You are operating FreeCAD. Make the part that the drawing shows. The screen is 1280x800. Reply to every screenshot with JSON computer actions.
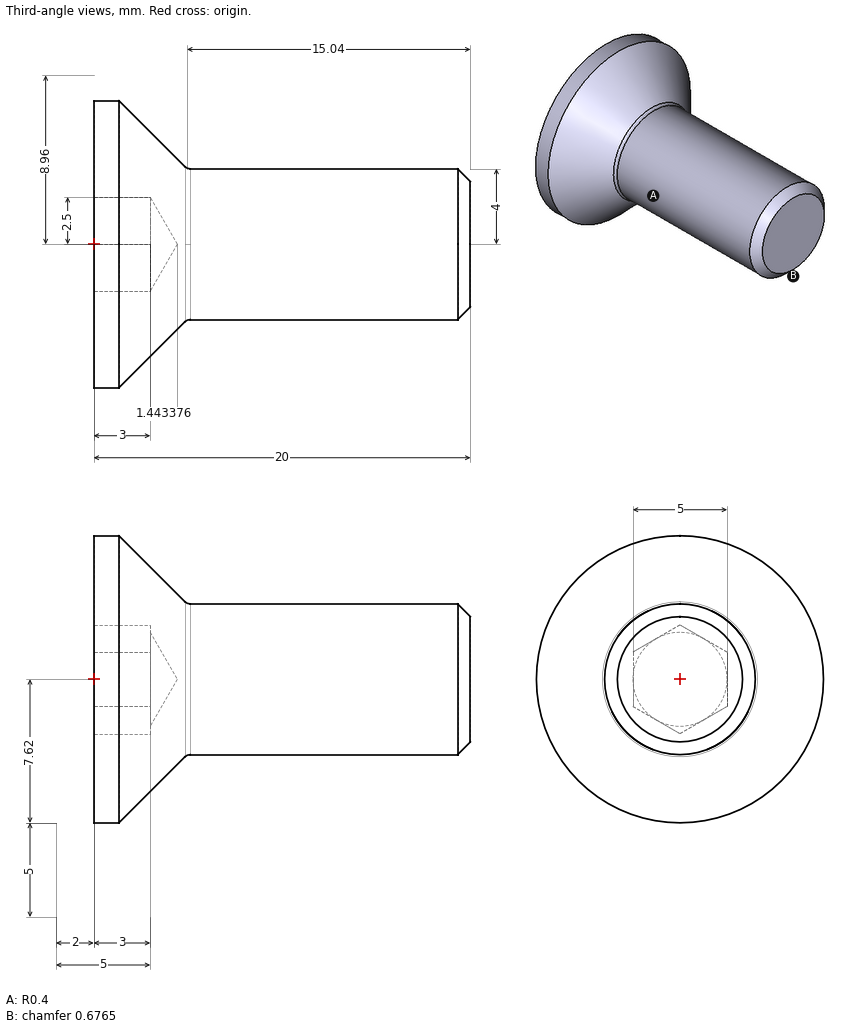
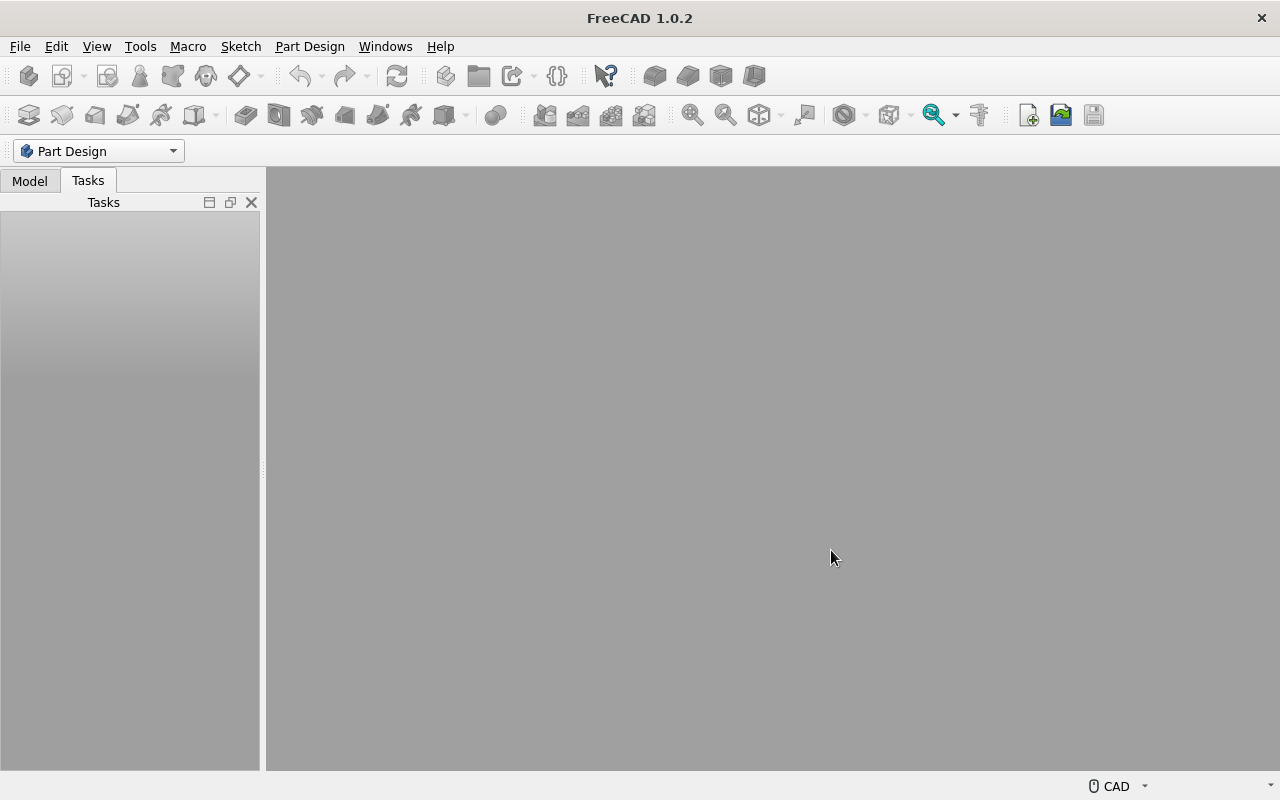
{"action": "left_click", "coordinate": [1028, 116]}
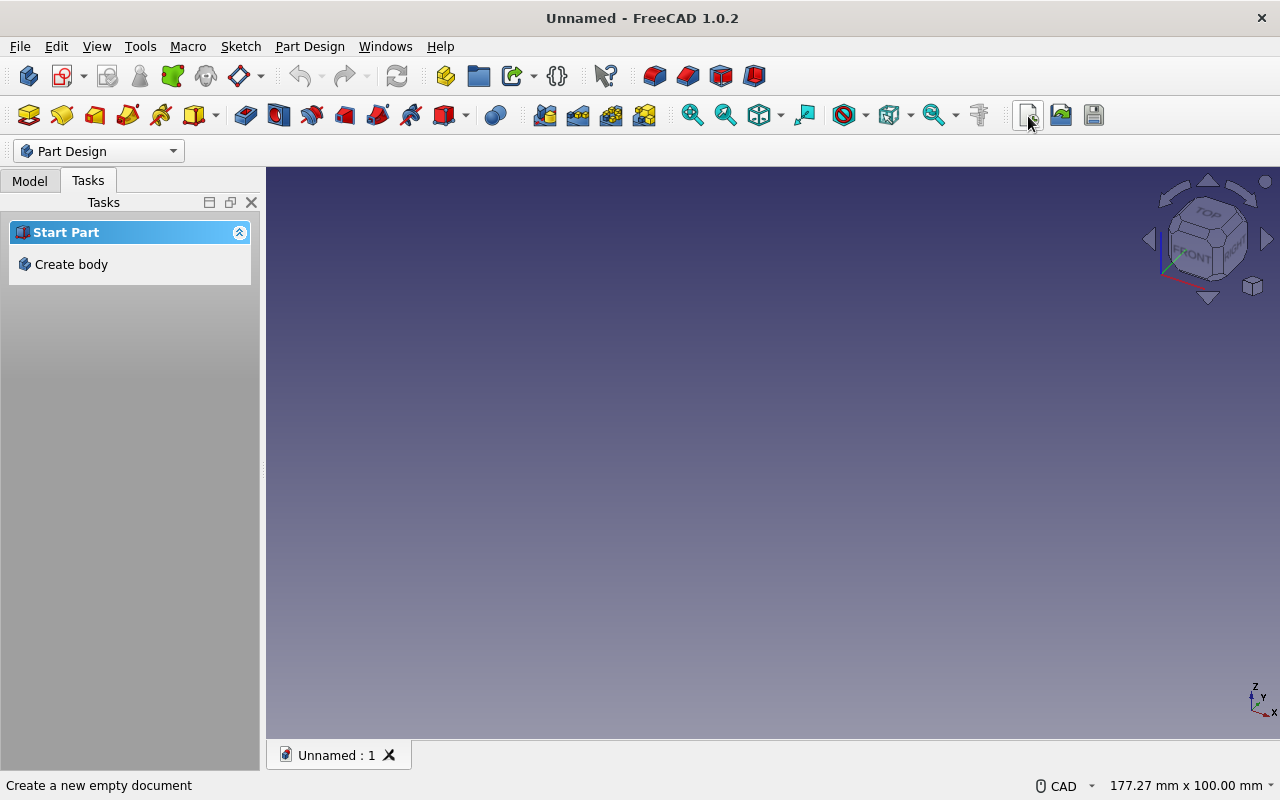
{"action": "left_click", "coordinate": [62, 76]}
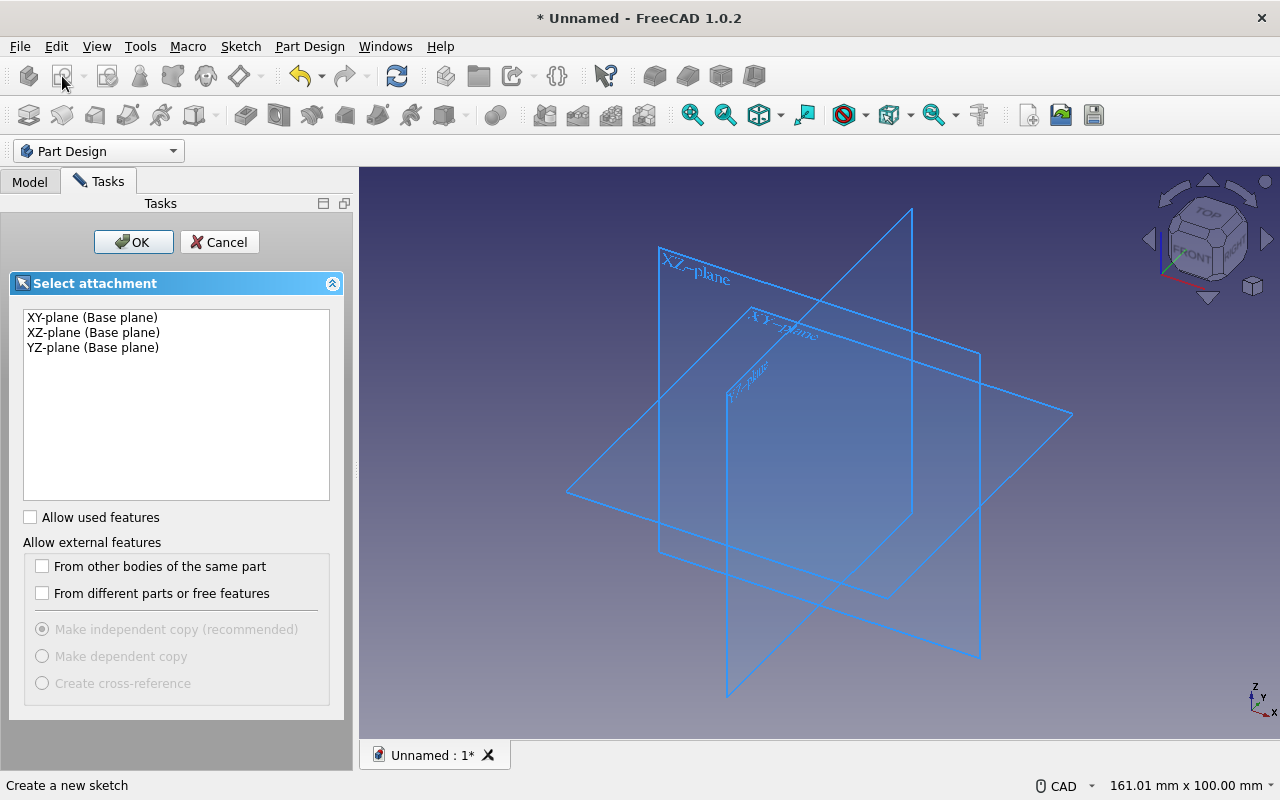
{"action": "left_click", "coordinate": [84, 318]}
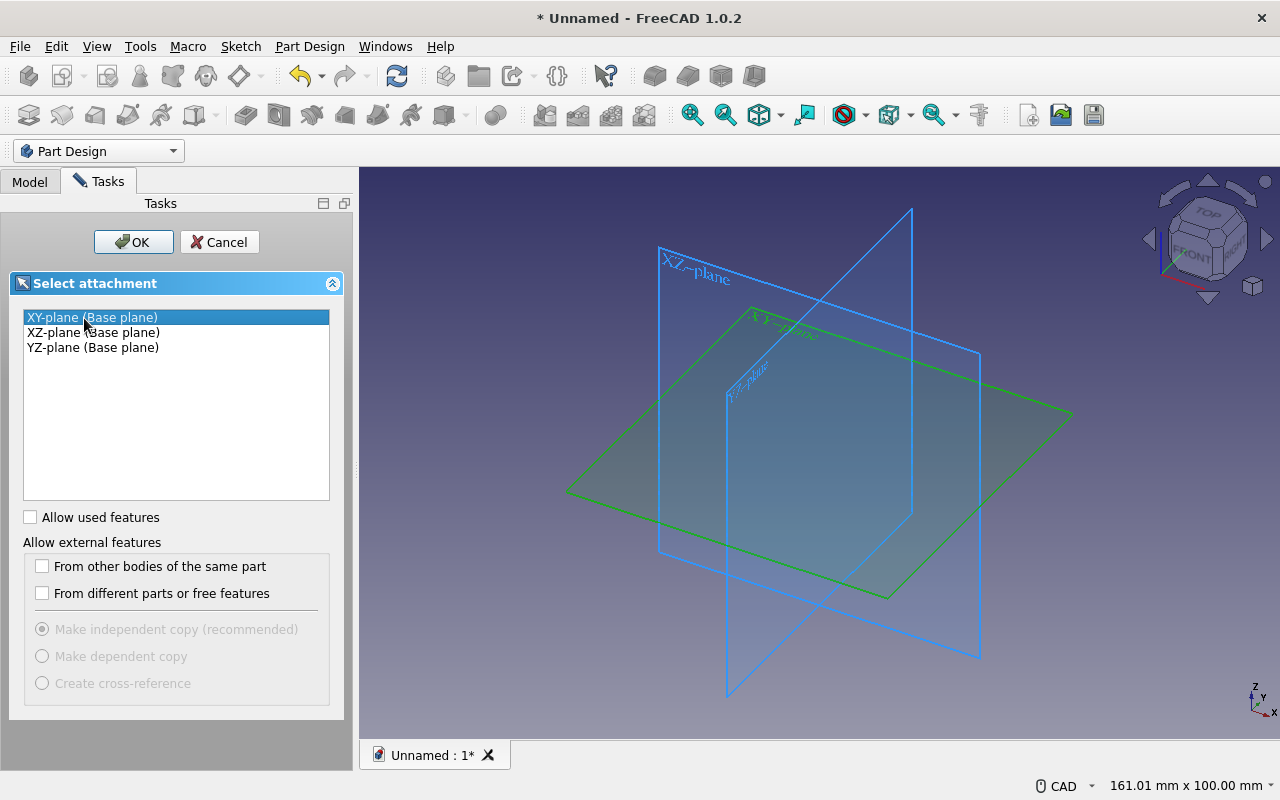
{"action": "left_click", "coordinate": [134, 242]}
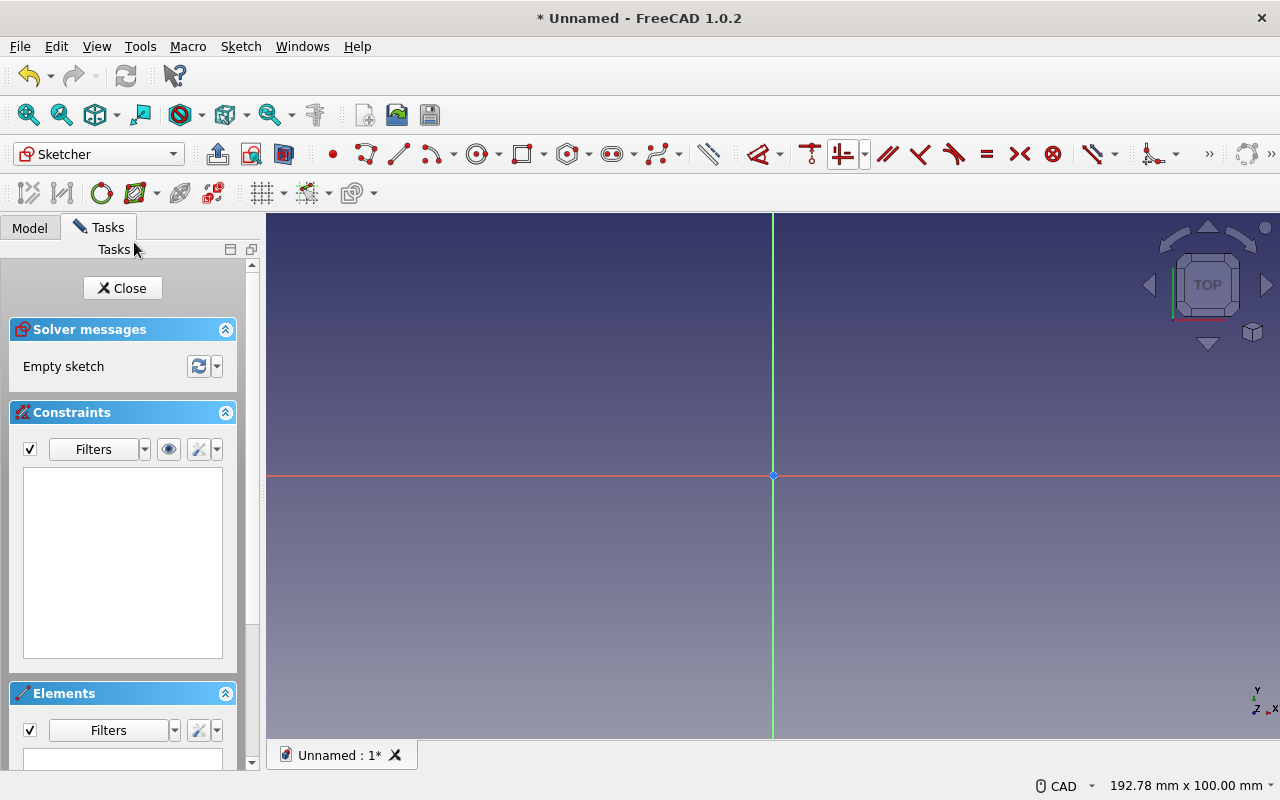
{"action": "scroll", "coordinate": [850, 448], "scroll_direction": "up", "scroll_amount": 9}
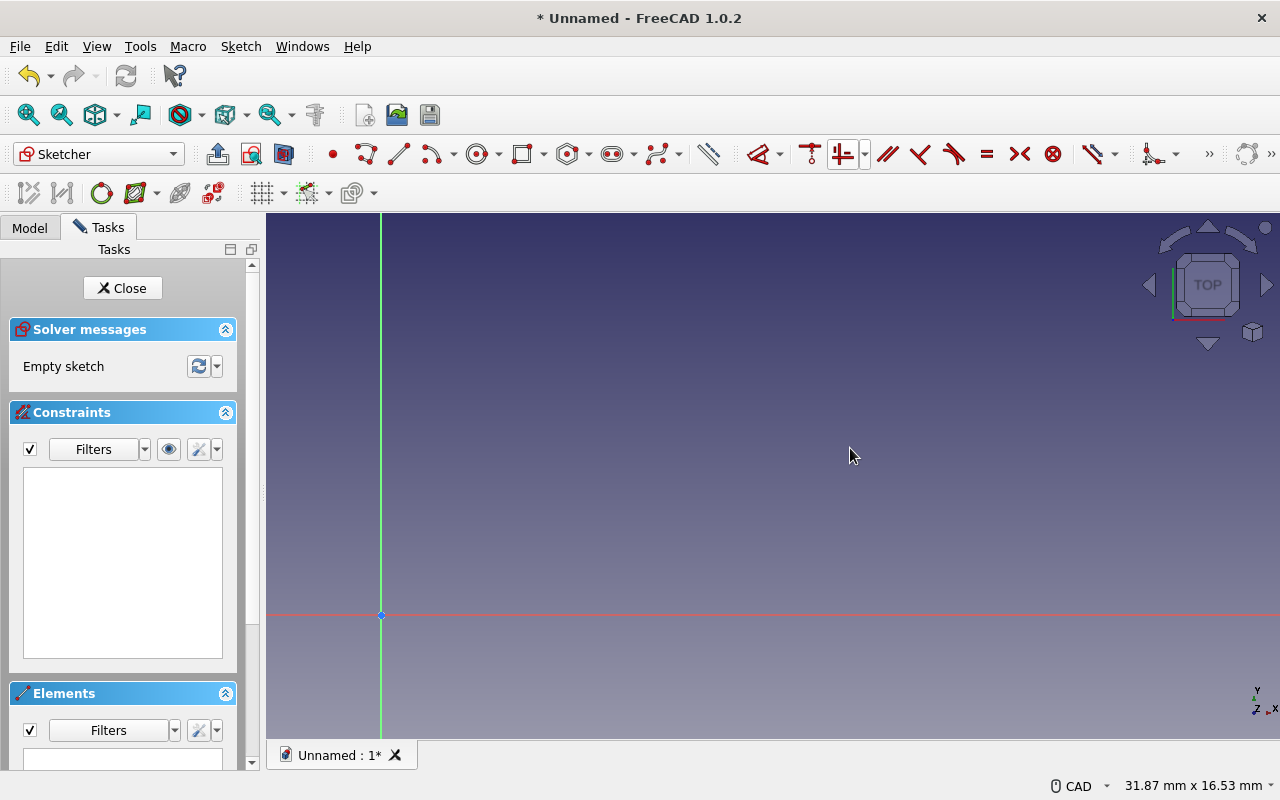
{"action": "left_click", "coordinate": [366, 154]}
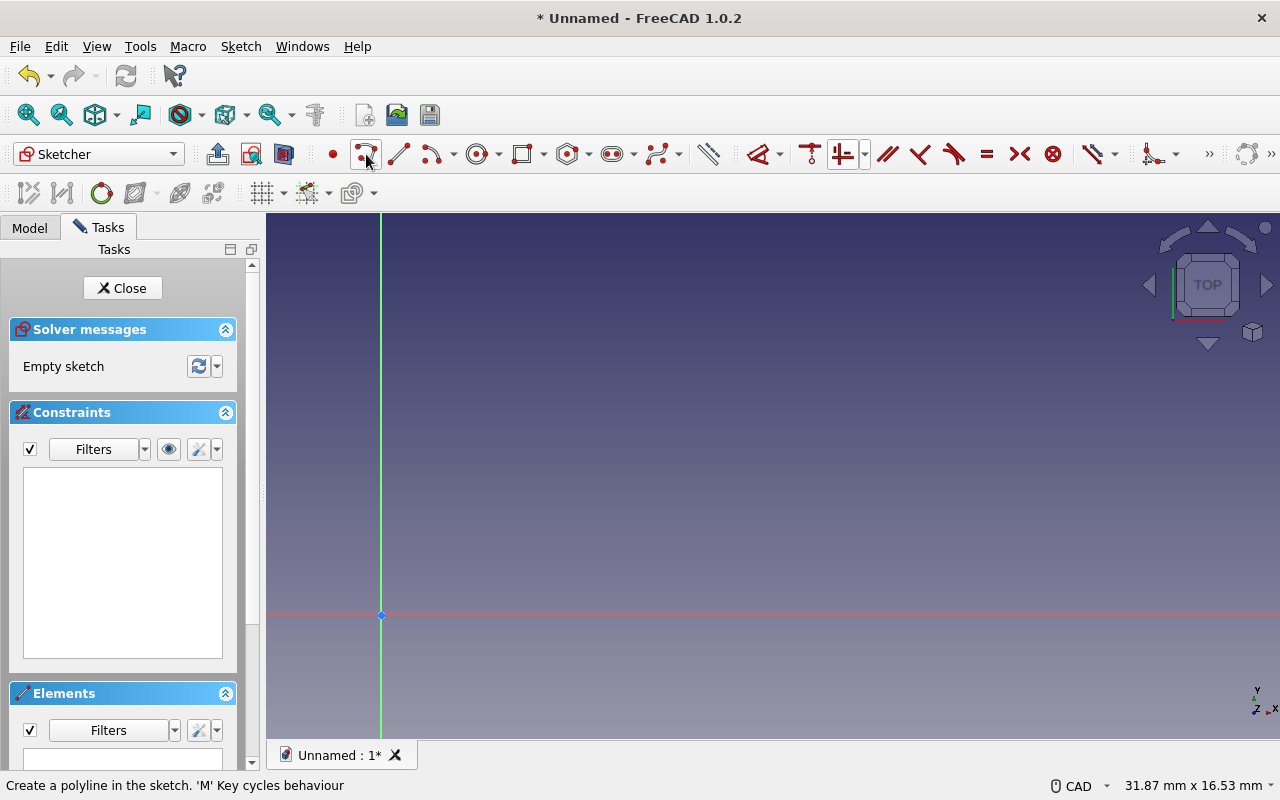
{"action": "left_click", "coordinate": [381, 615]}
{"action": "left_click", "coordinate": [1018, 606]}
{"action": "left_click", "coordinate": [1018, 488]}
{"action": "left_click", "coordinate": [539, 488]}
{"action": "left_click", "coordinate": [390, 330]}
{"action": "left_click", "coordinate": [381, 615]}
{"action": "key", "text": "Escape"}
{"action": "key", "text": "Escape"}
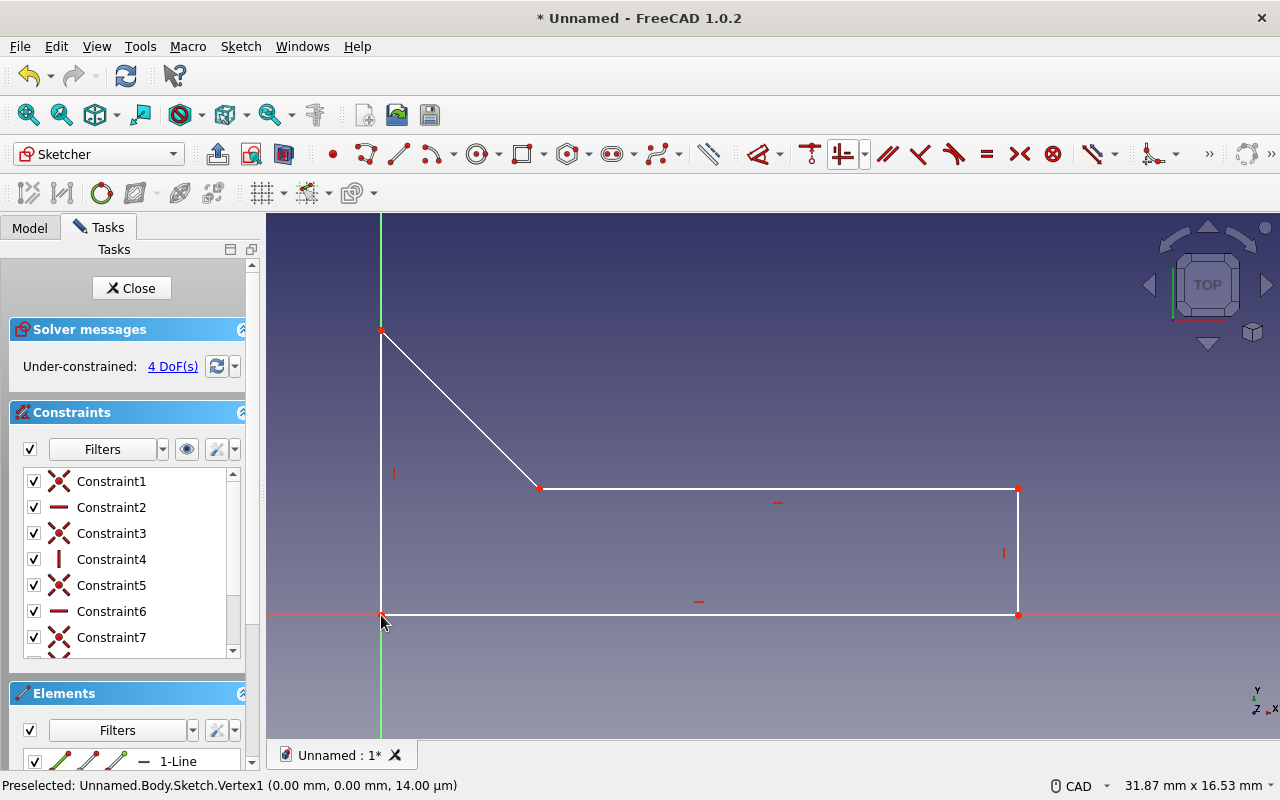
{"action": "left_click", "coordinate": [758, 154]}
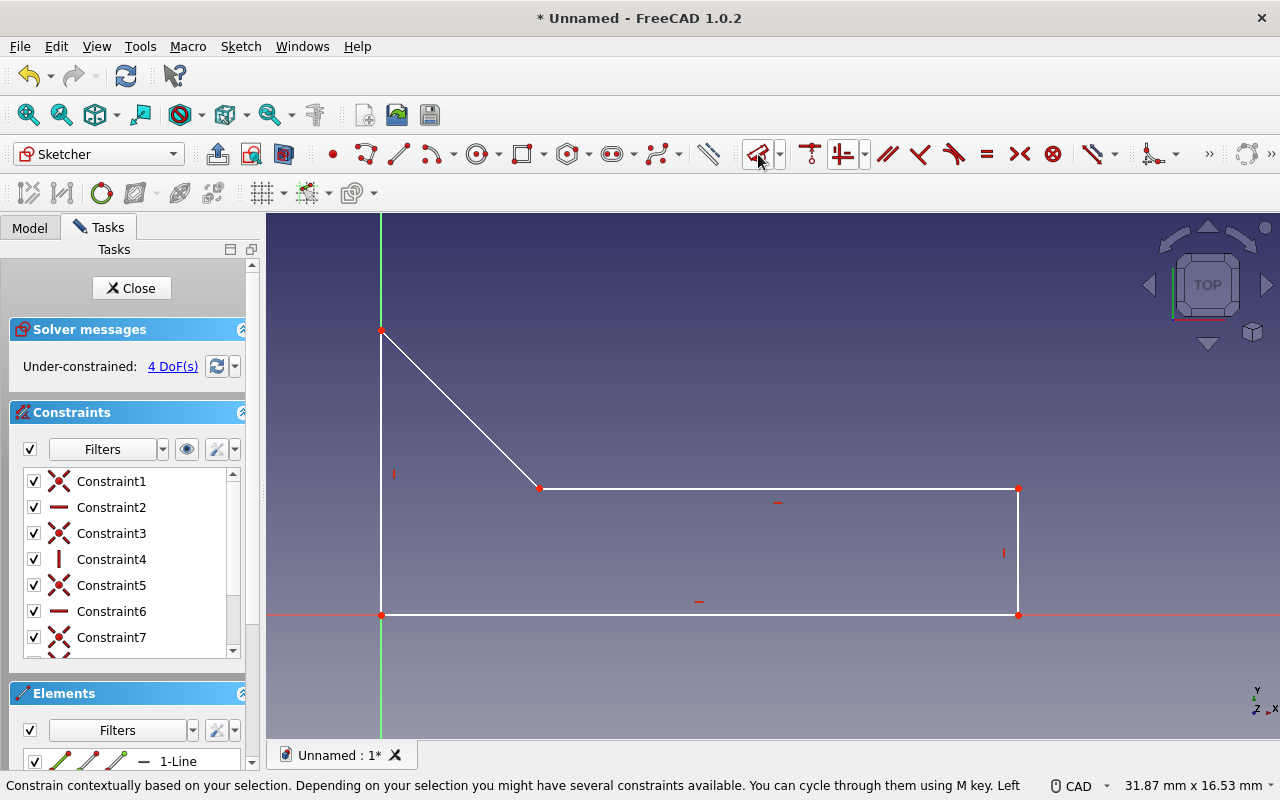
{"action": "left_click", "coordinate": [1018, 577]}
{"action": "left_click", "coordinate": [1052, 552]}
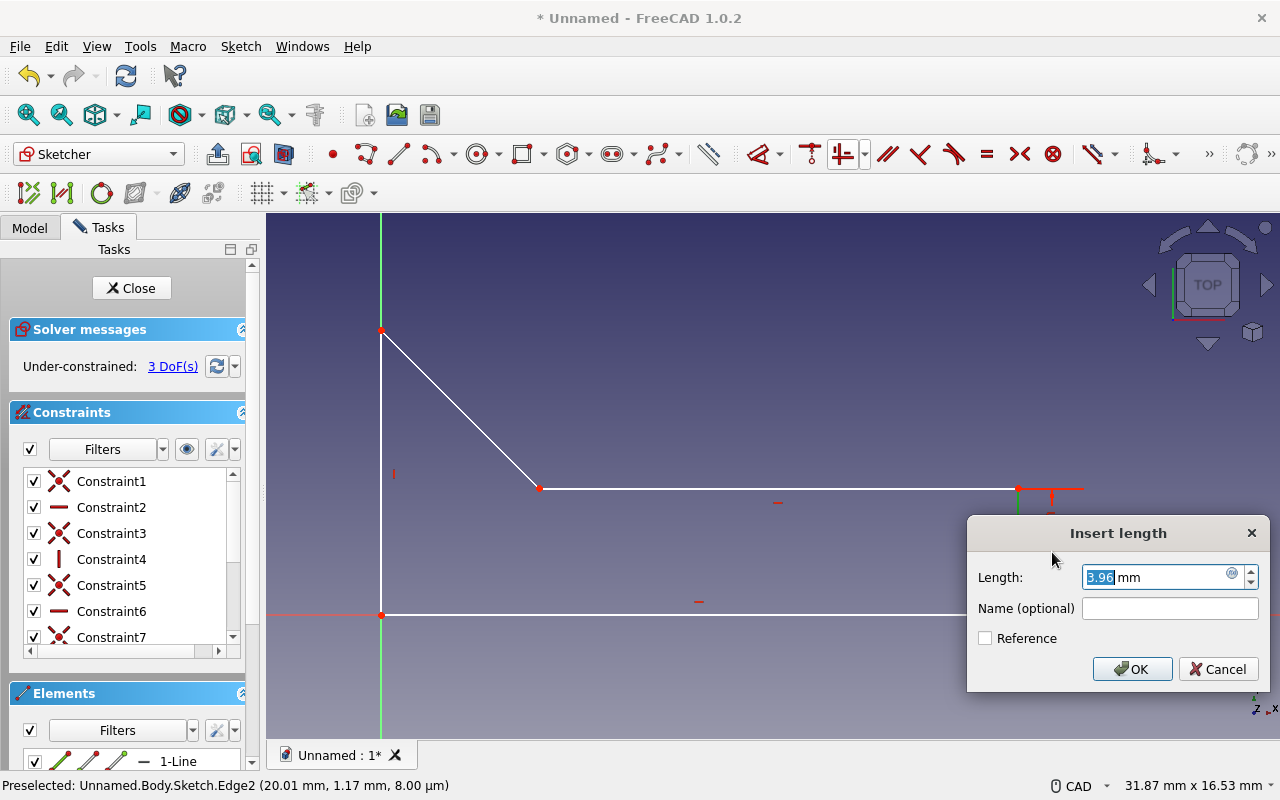
{"action": "type", "text": "4"}
{"action": "key", "text": "Return"}